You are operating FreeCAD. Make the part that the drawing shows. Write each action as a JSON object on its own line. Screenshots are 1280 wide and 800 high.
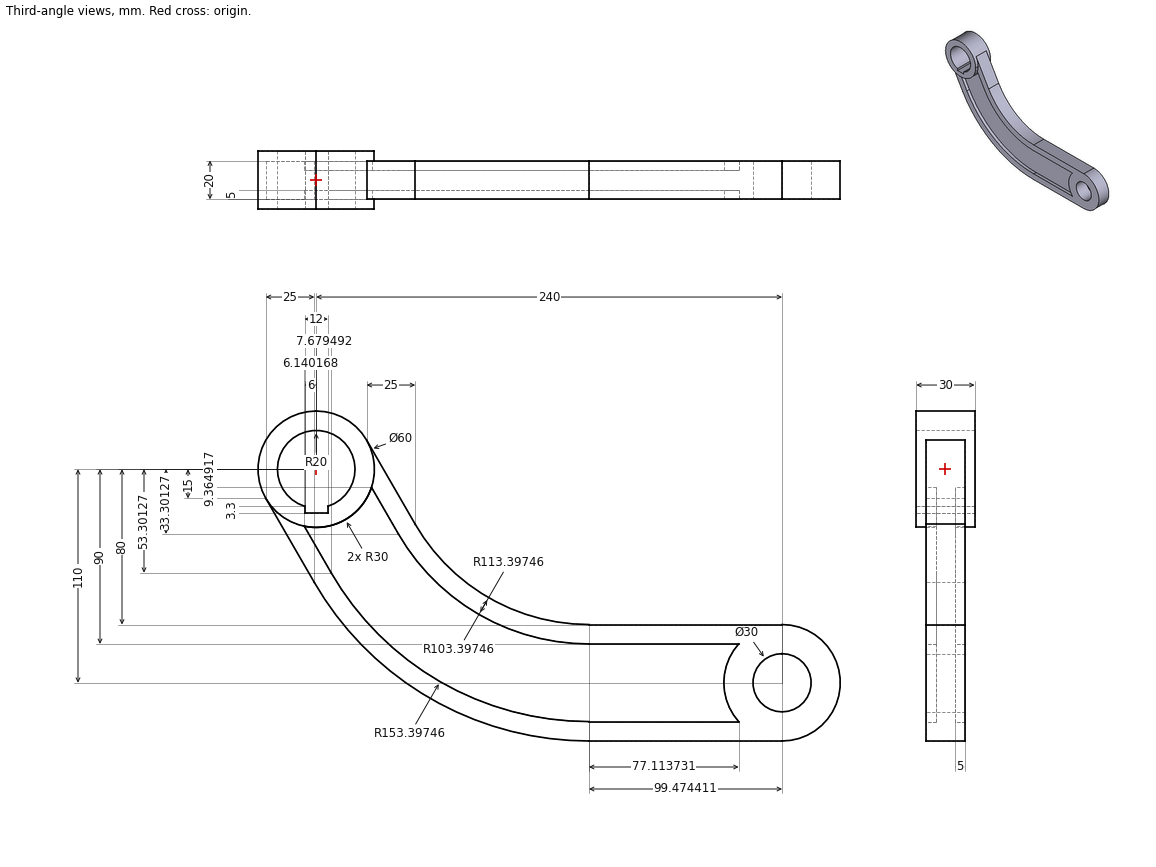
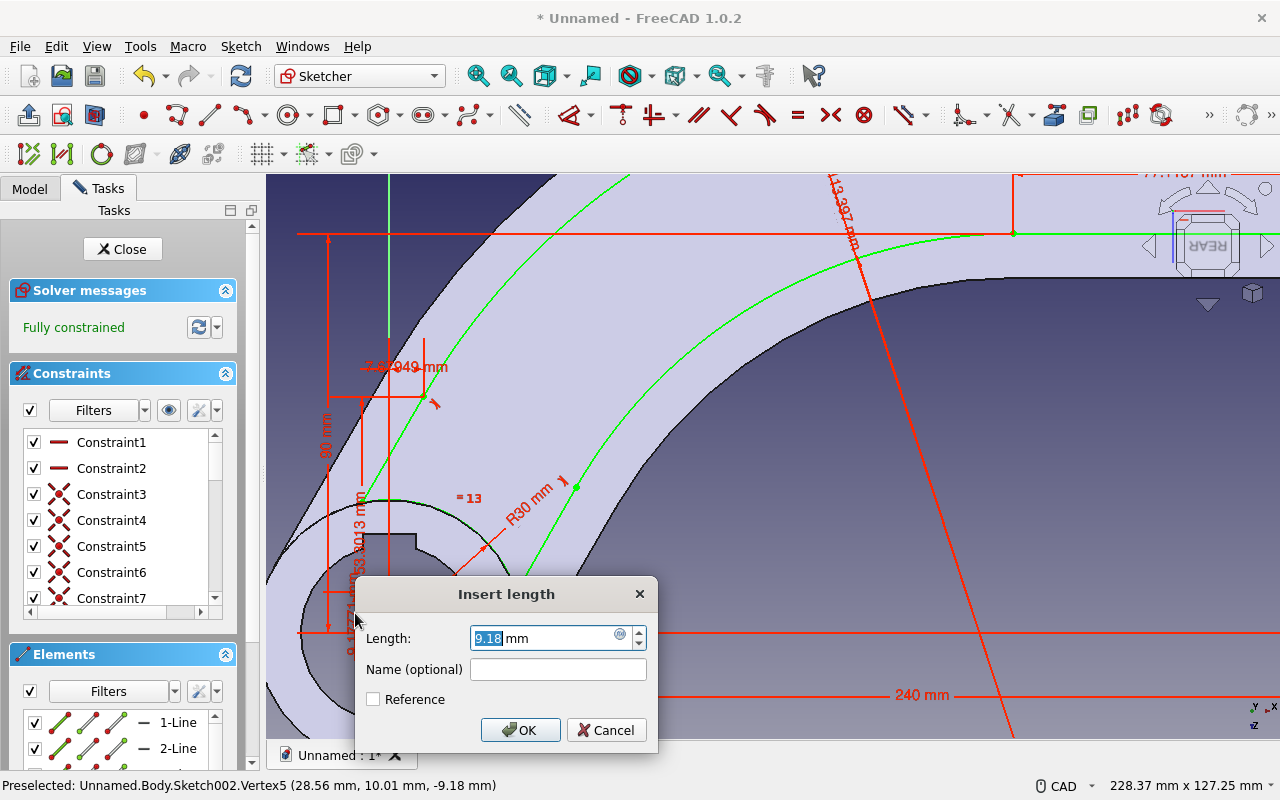
{"action": "type", "text": "9.364917"}
{"action": "key", "text": "Return"}
{"action": "key", "text": "Escape"}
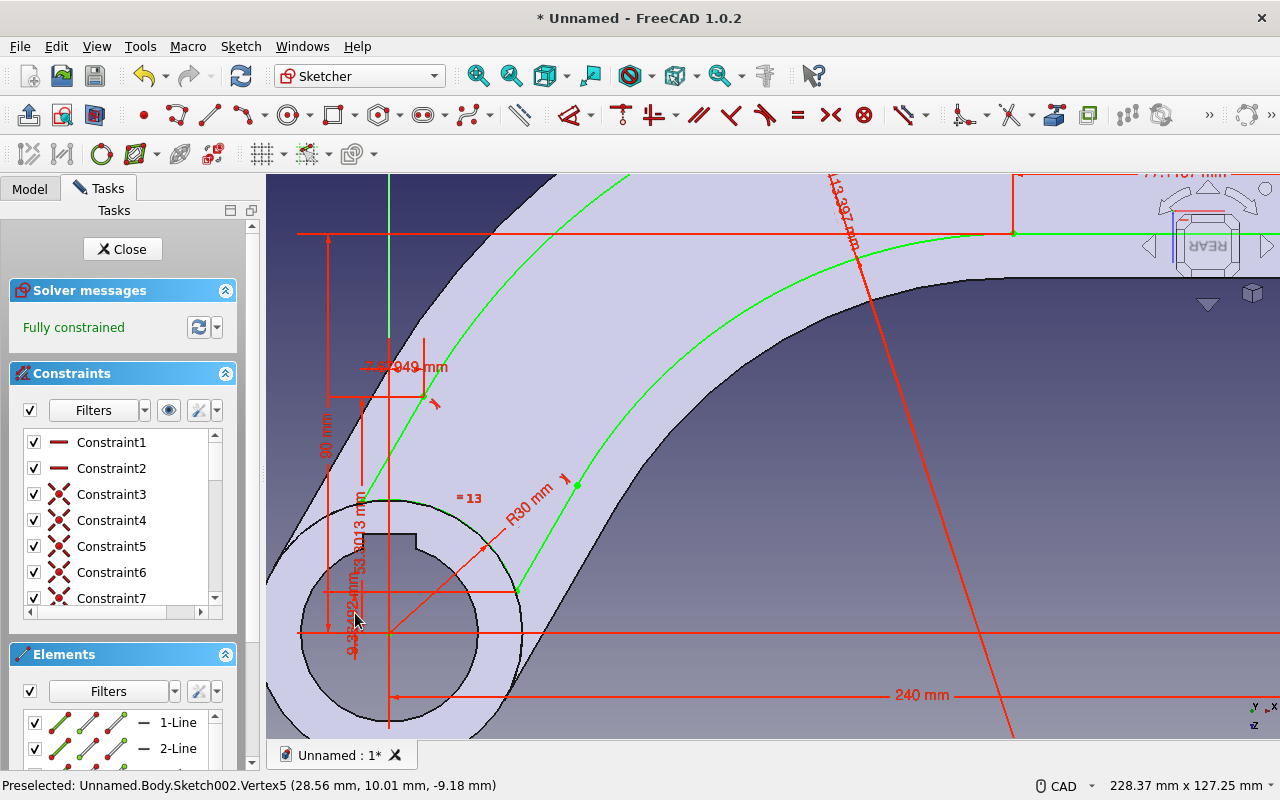
{"action": "left_click", "coordinate": [123, 249]}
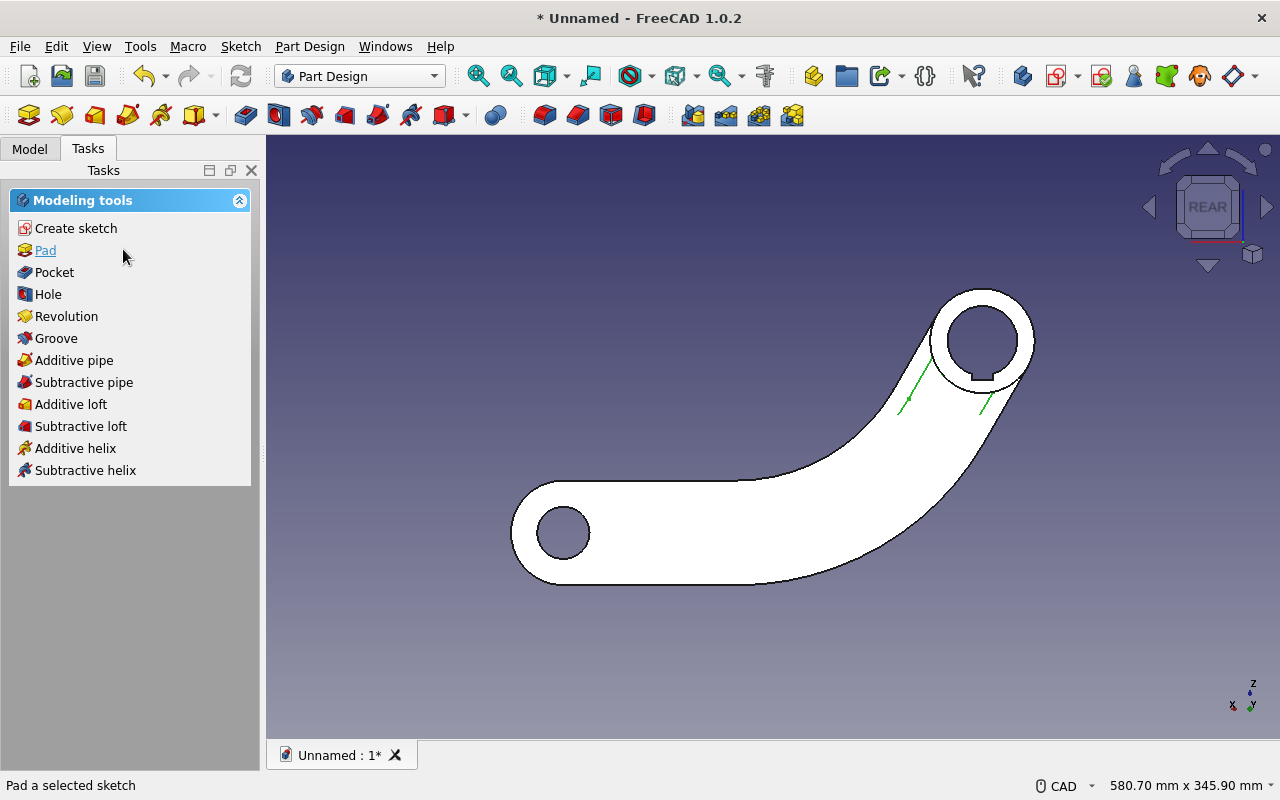
{"action": "left_click", "coordinate": [246, 116]}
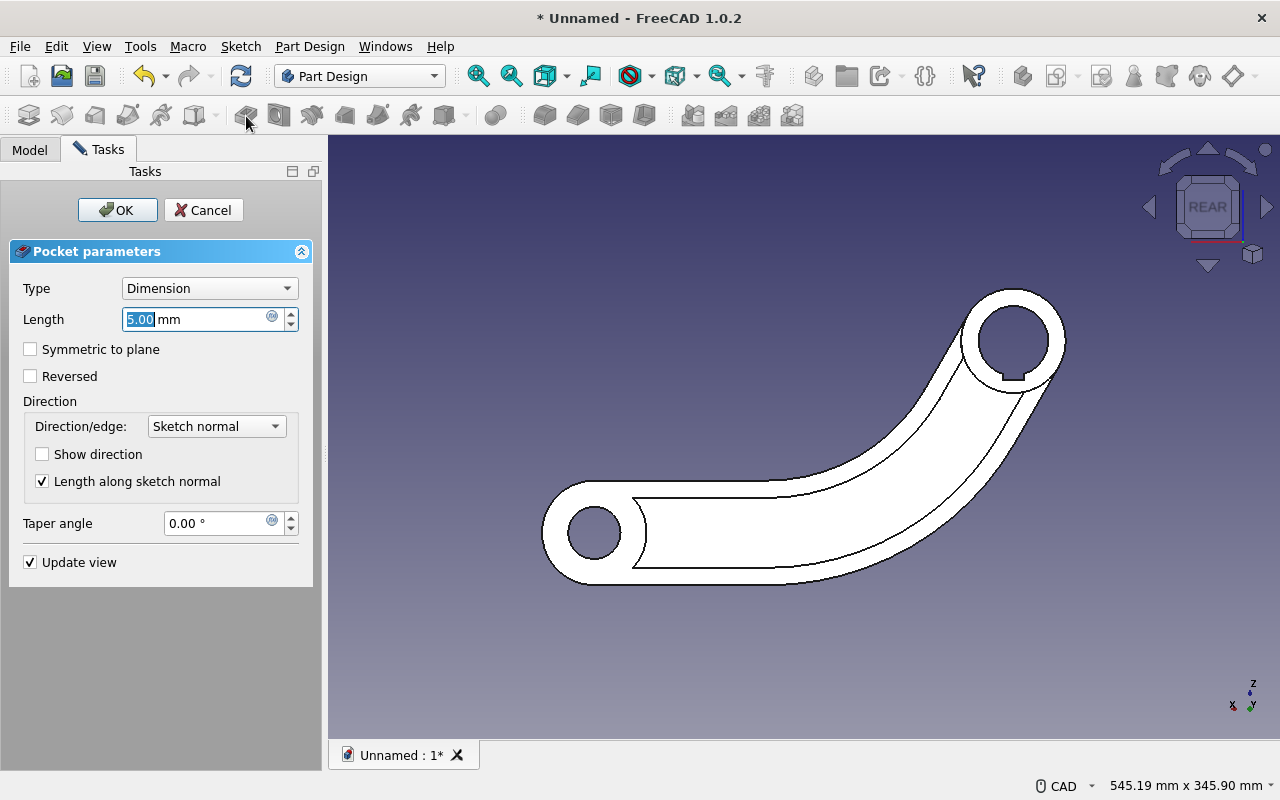
{"action": "type", "text": "5"}
{"action": "key", "text": "Tab"}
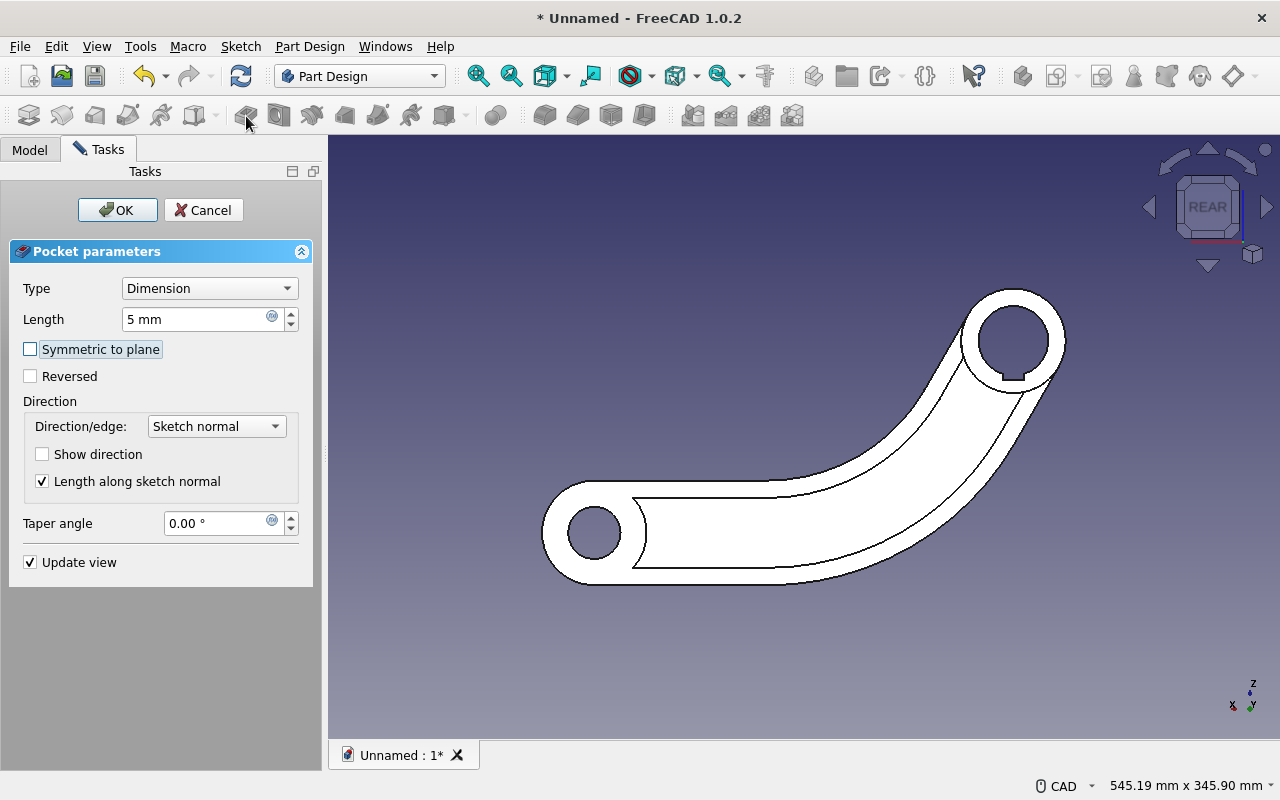
{"action": "left_click", "coordinate": [118, 210]}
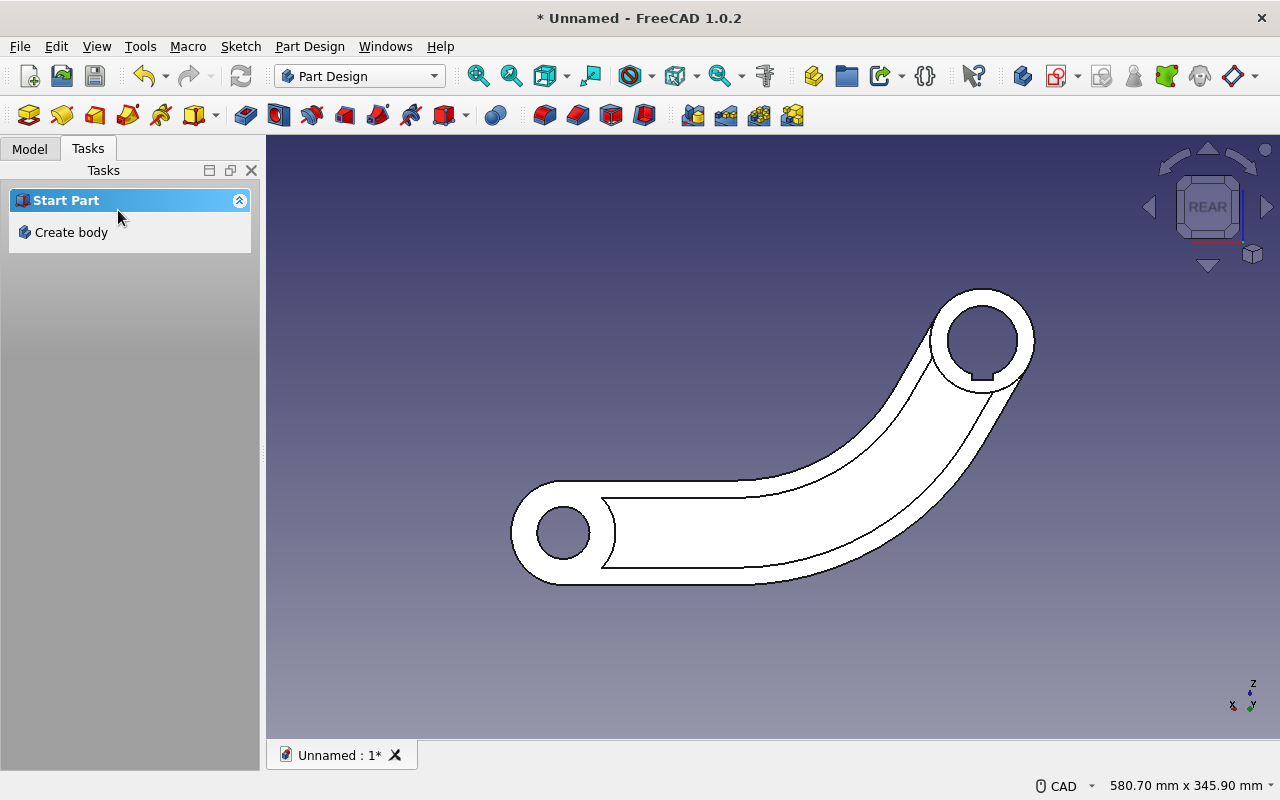
{"action": "left_click", "coordinate": [30, 148]}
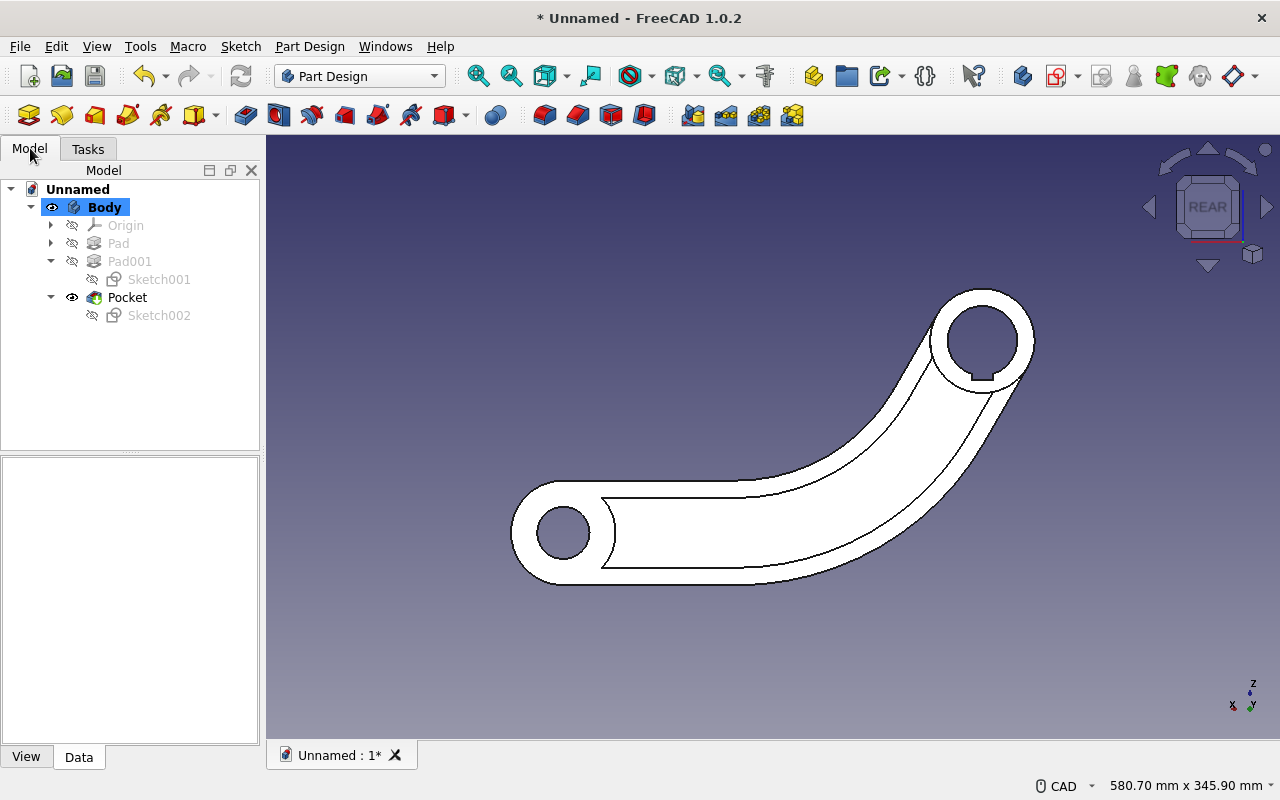
{"action": "left_click", "coordinate": [51, 225]}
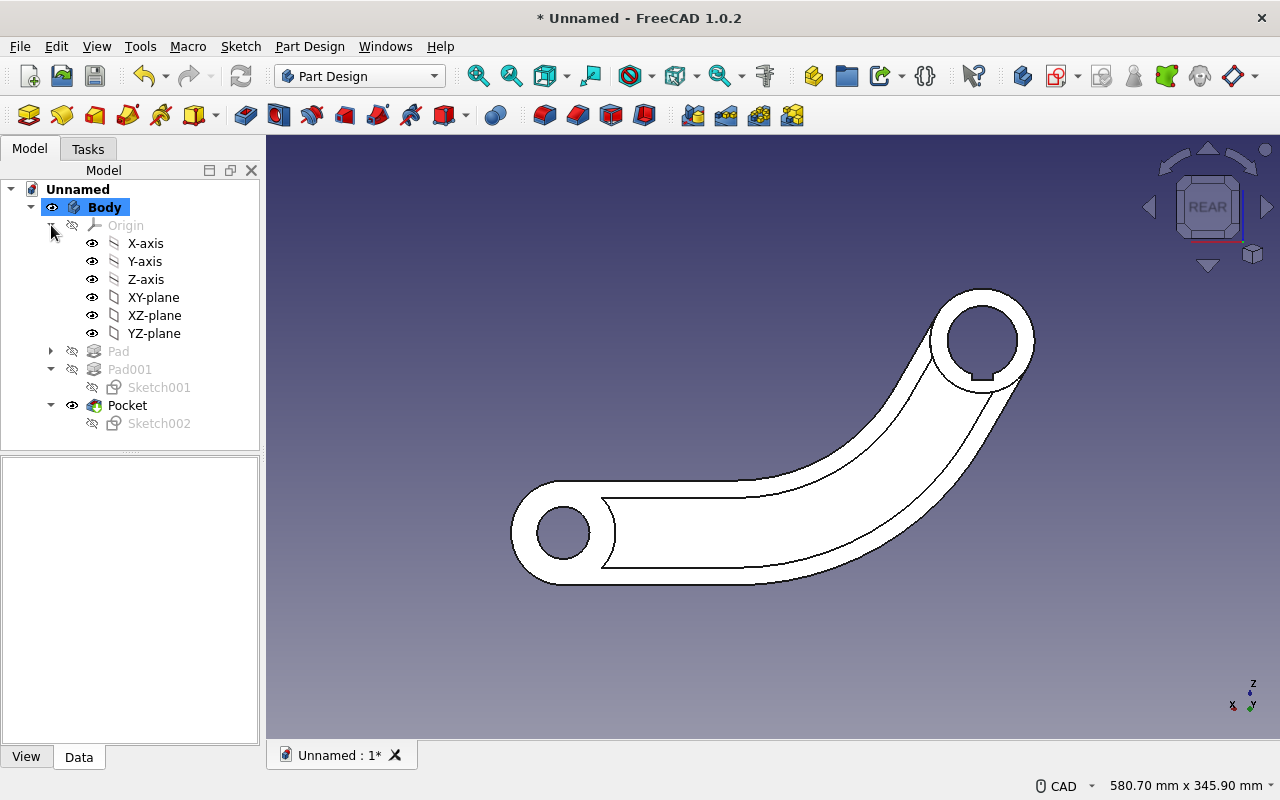
{"action": "left_click", "coordinate": [137, 315]}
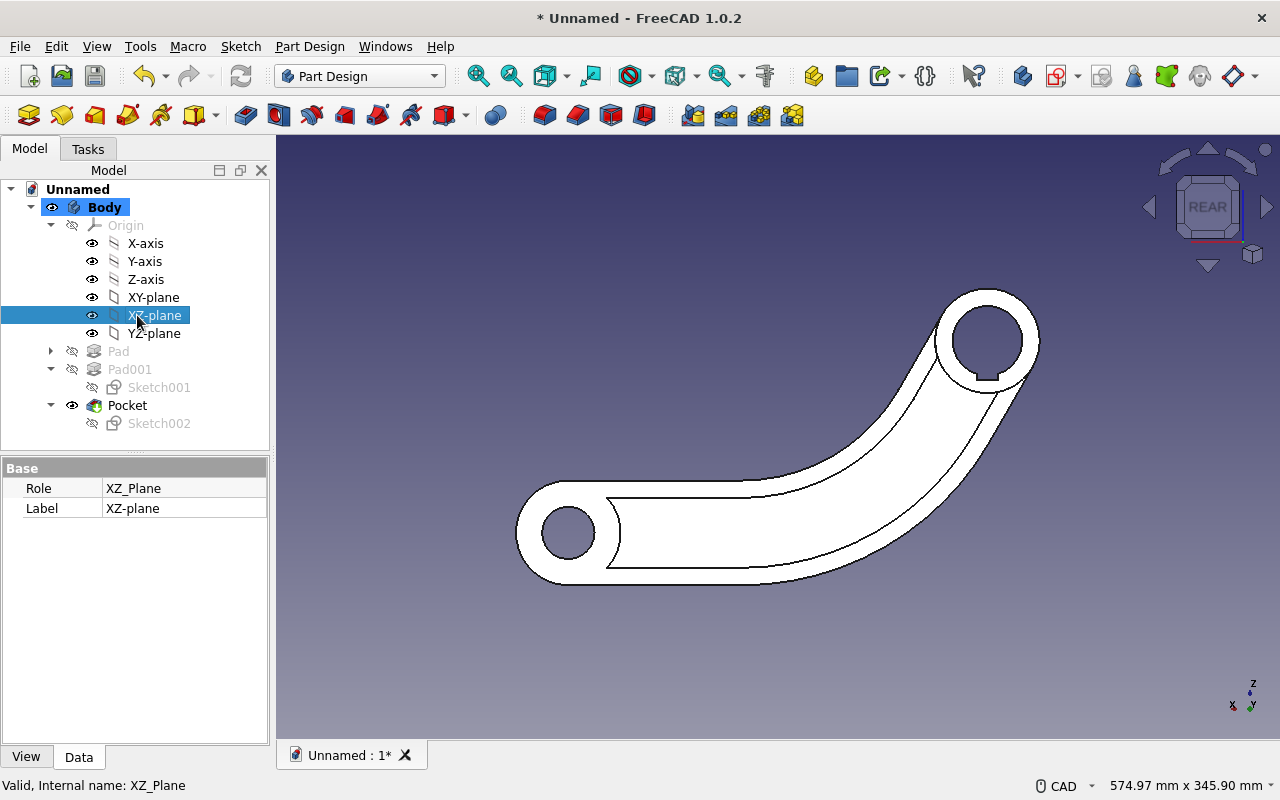
{"action": "left_click", "coordinate": [1232, 76]}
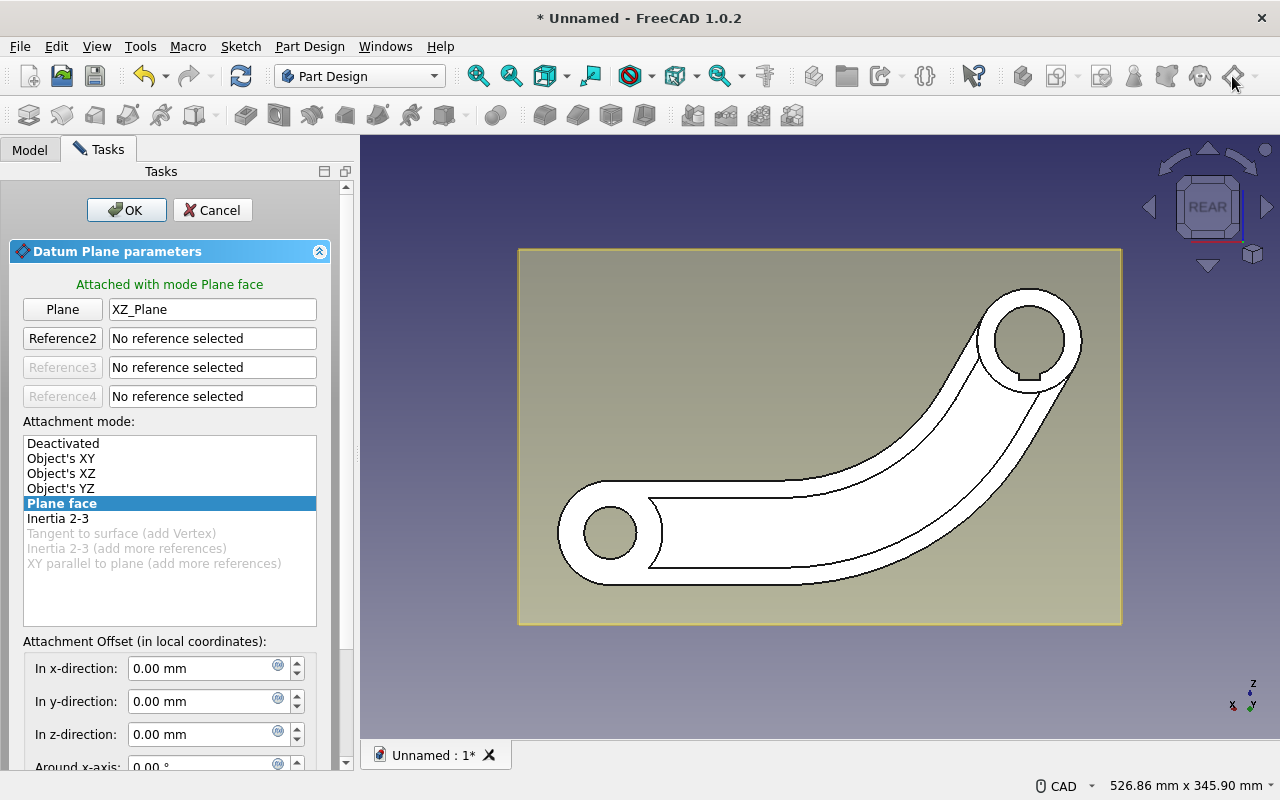
{"action": "triple_click", "coordinate": [210, 734]}